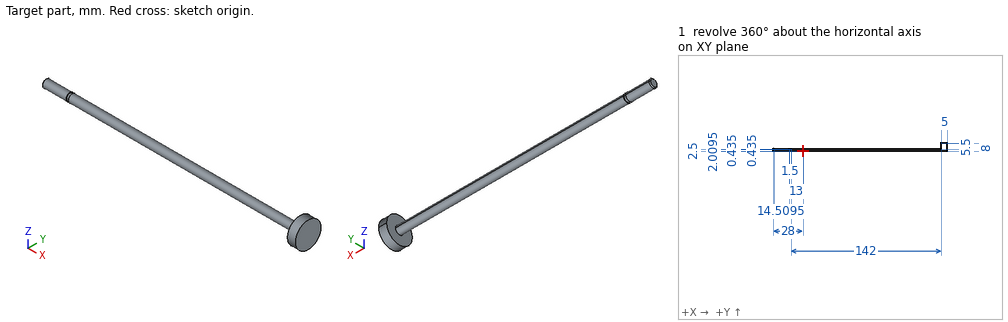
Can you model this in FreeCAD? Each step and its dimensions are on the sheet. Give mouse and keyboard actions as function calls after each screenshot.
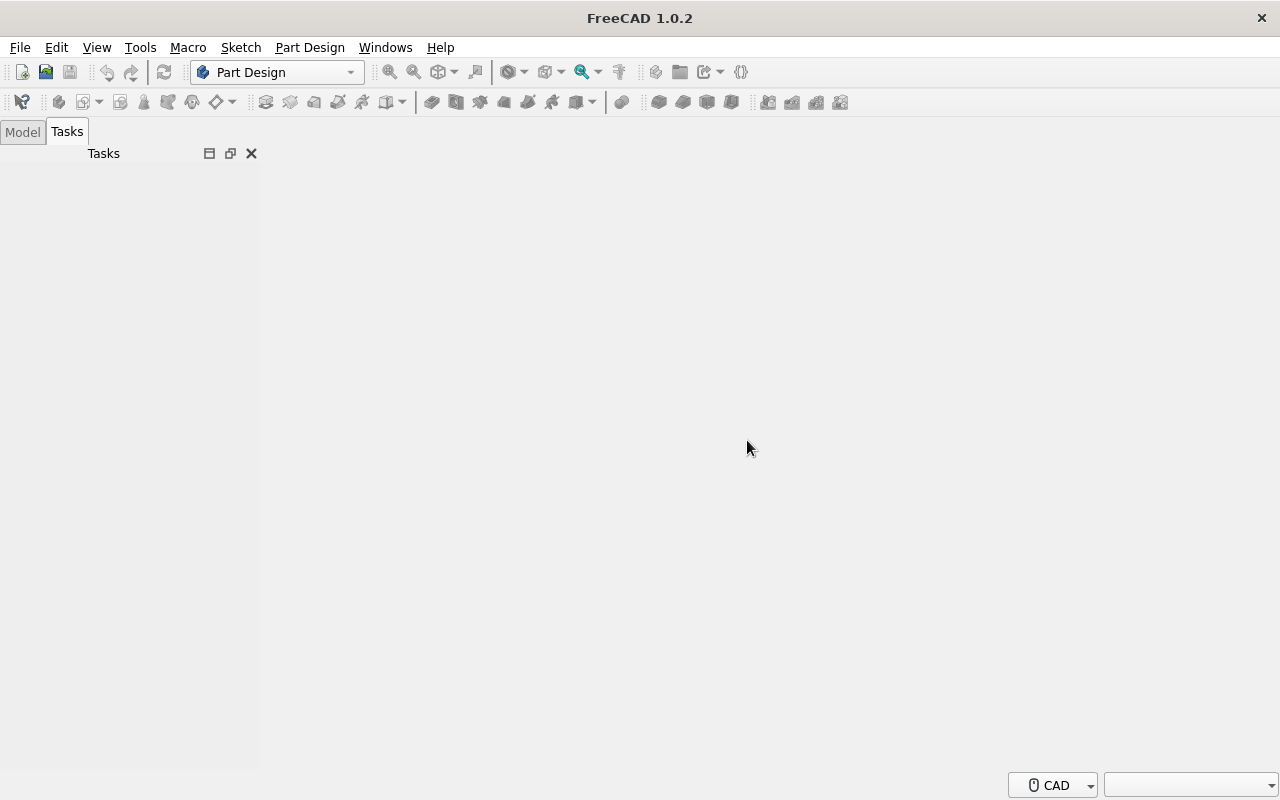
key(ctrl+n)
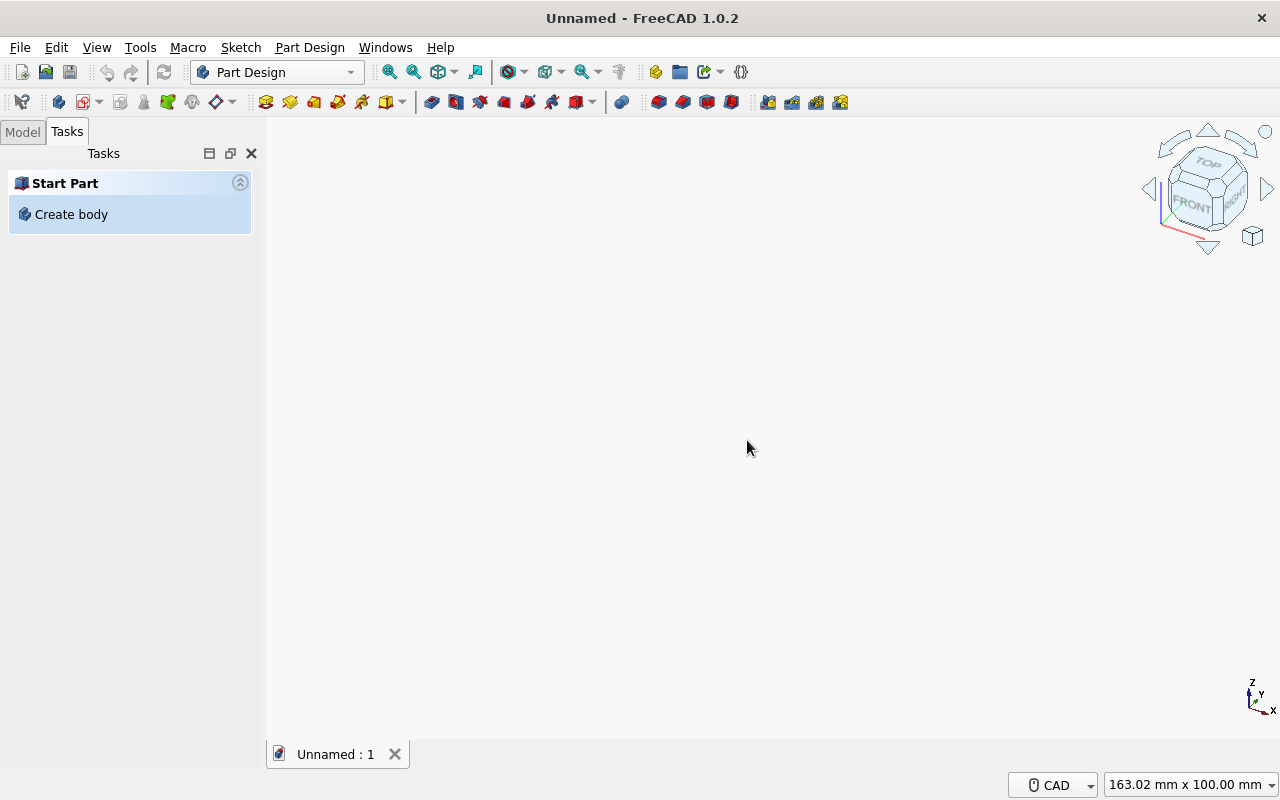
click(84, 102)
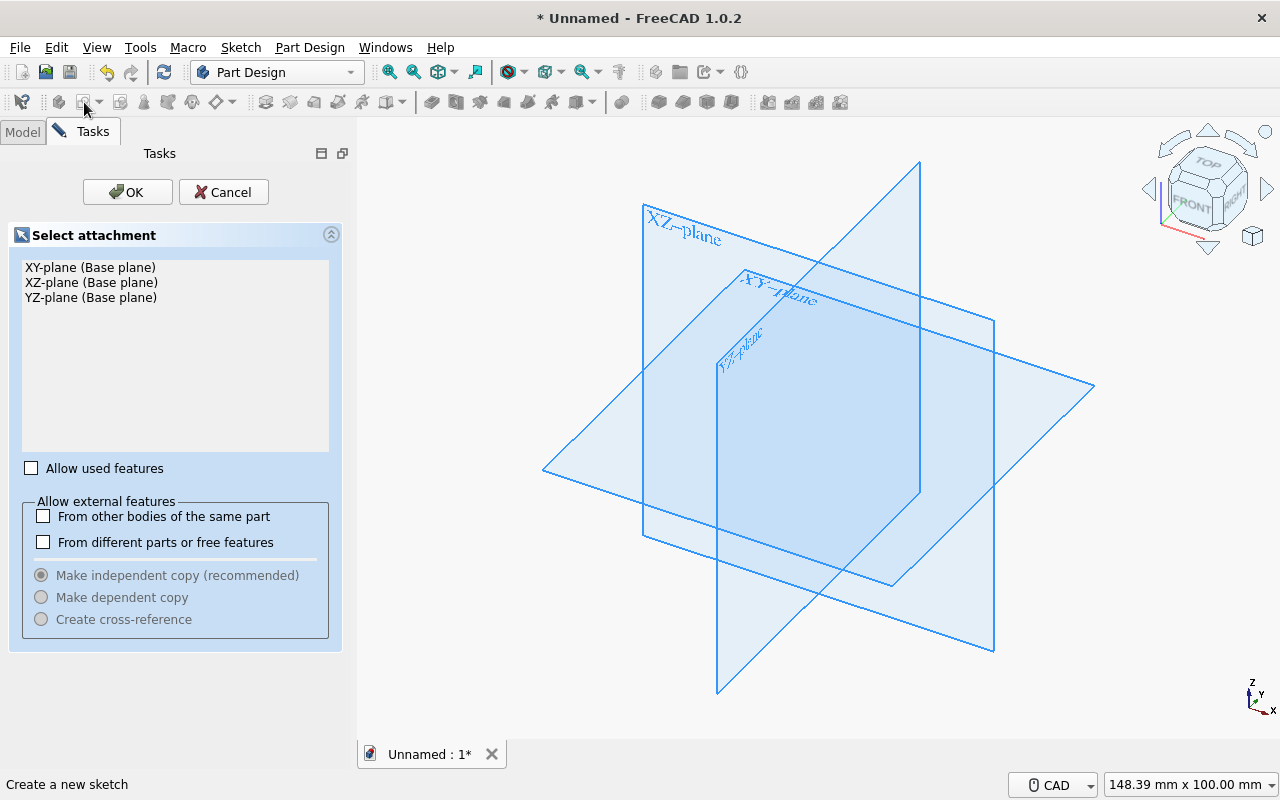
click(82, 268)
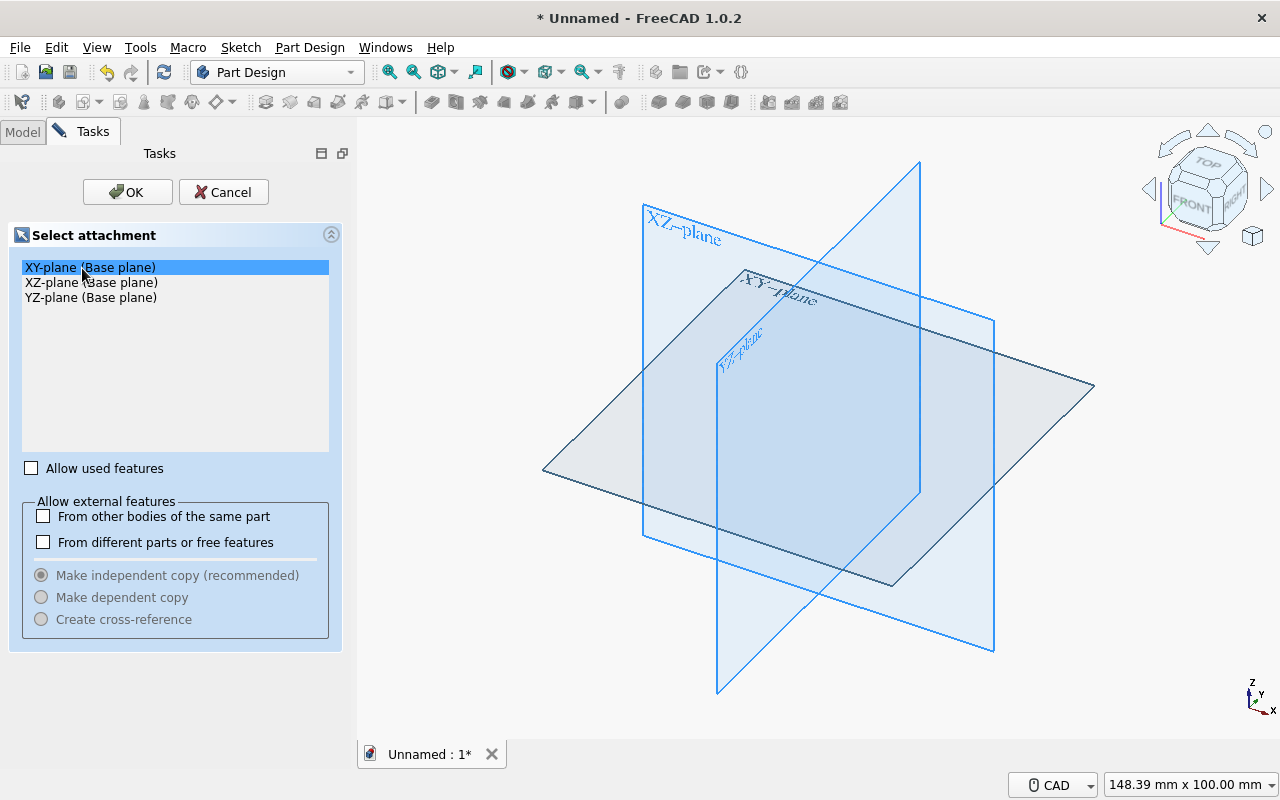
click(128, 192)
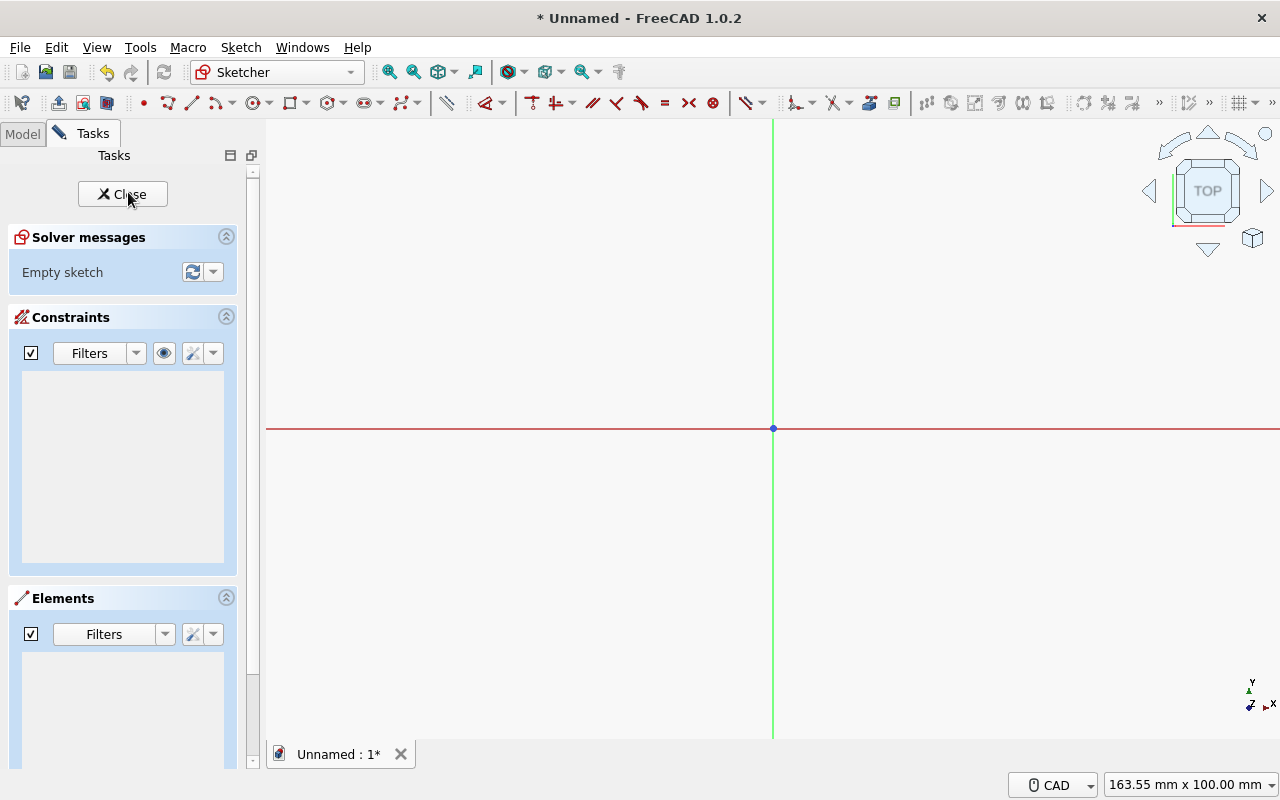
scroll(294, 459, down, 3)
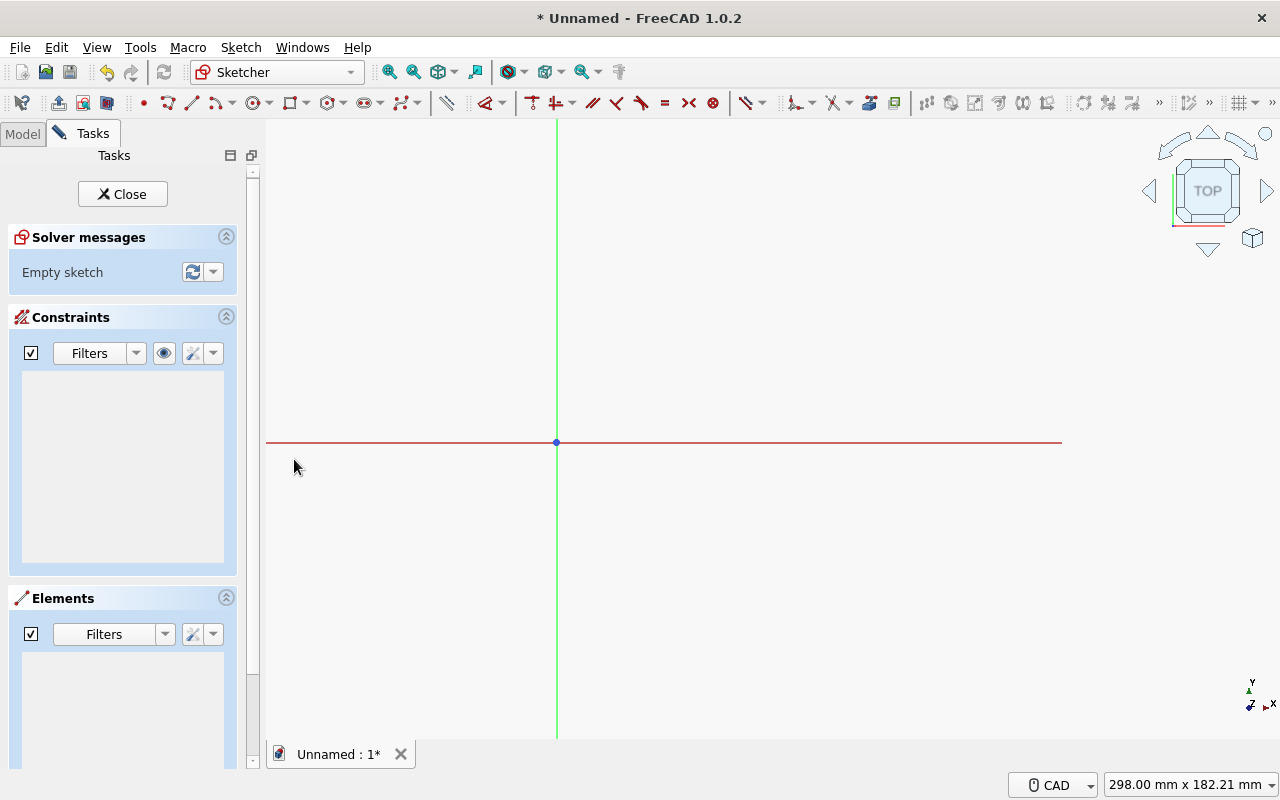
click(168, 104)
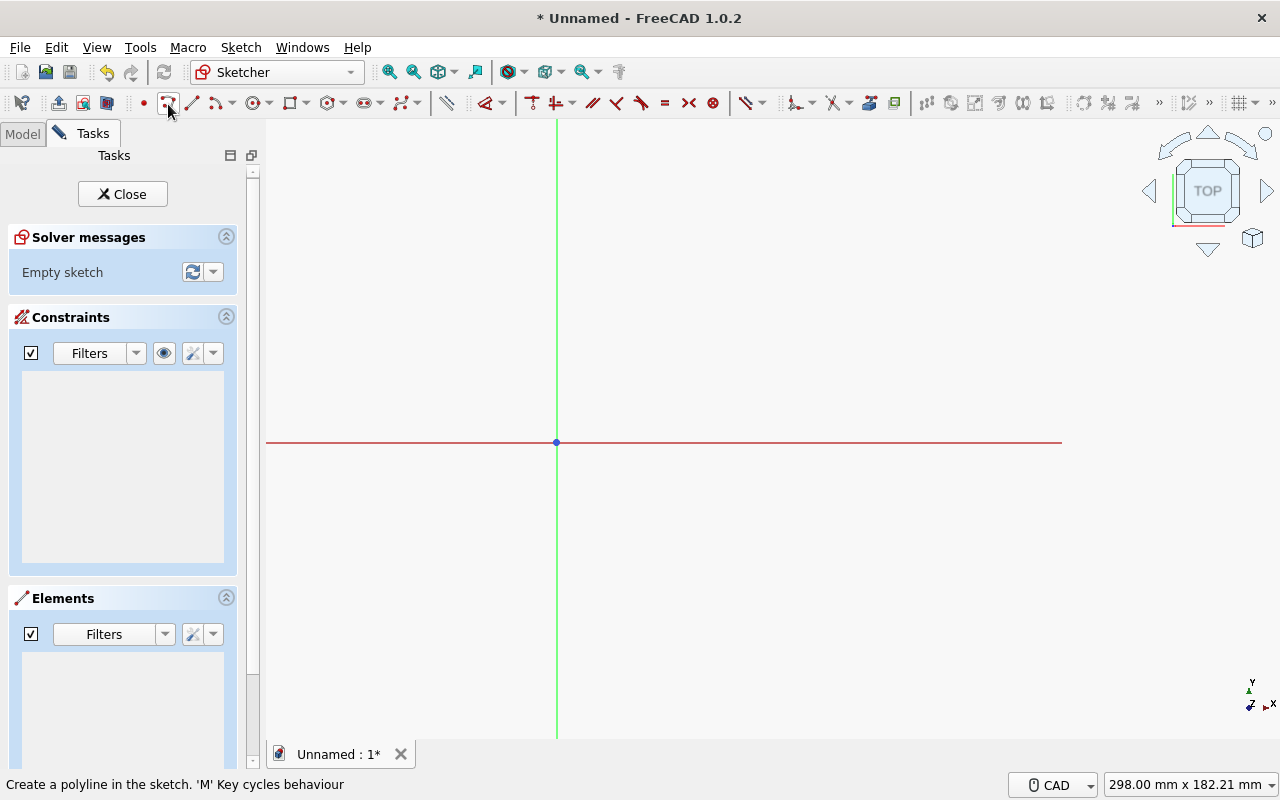
scroll(518, 436, up, 5)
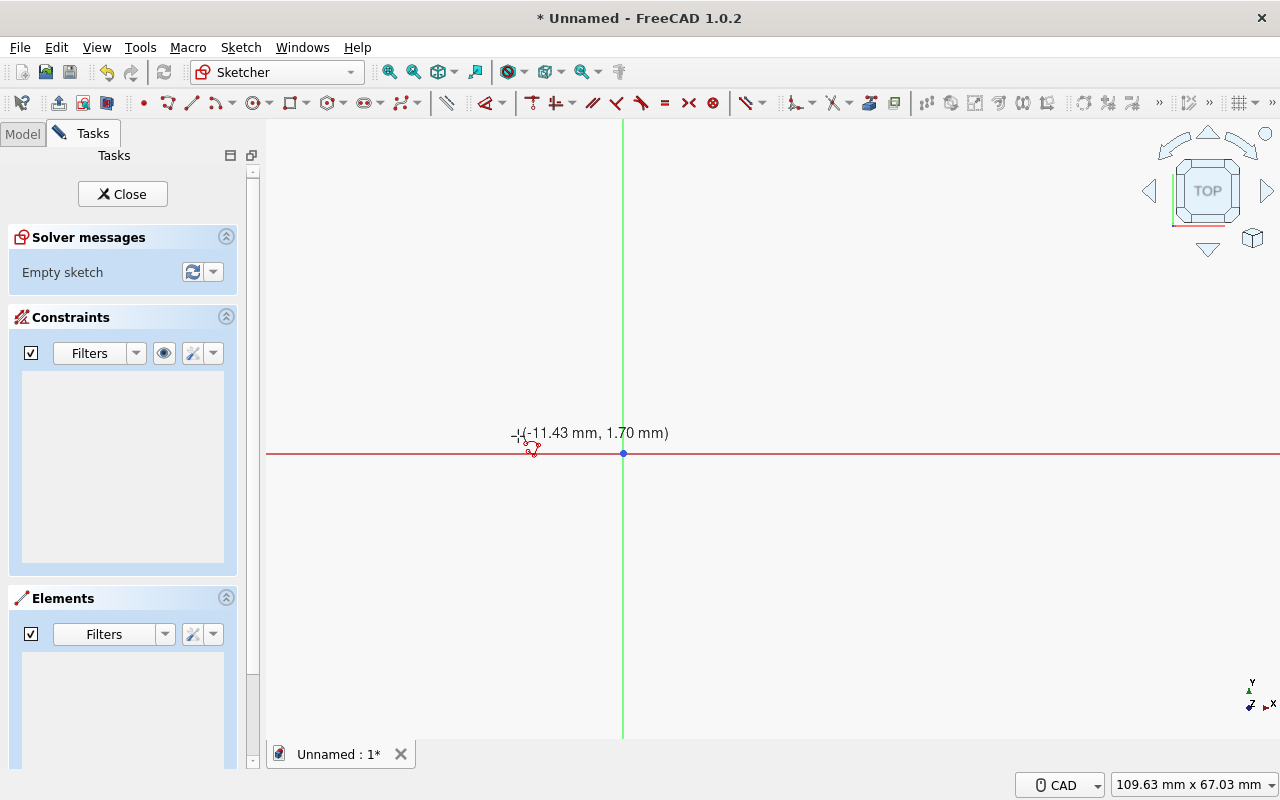
click(517, 434)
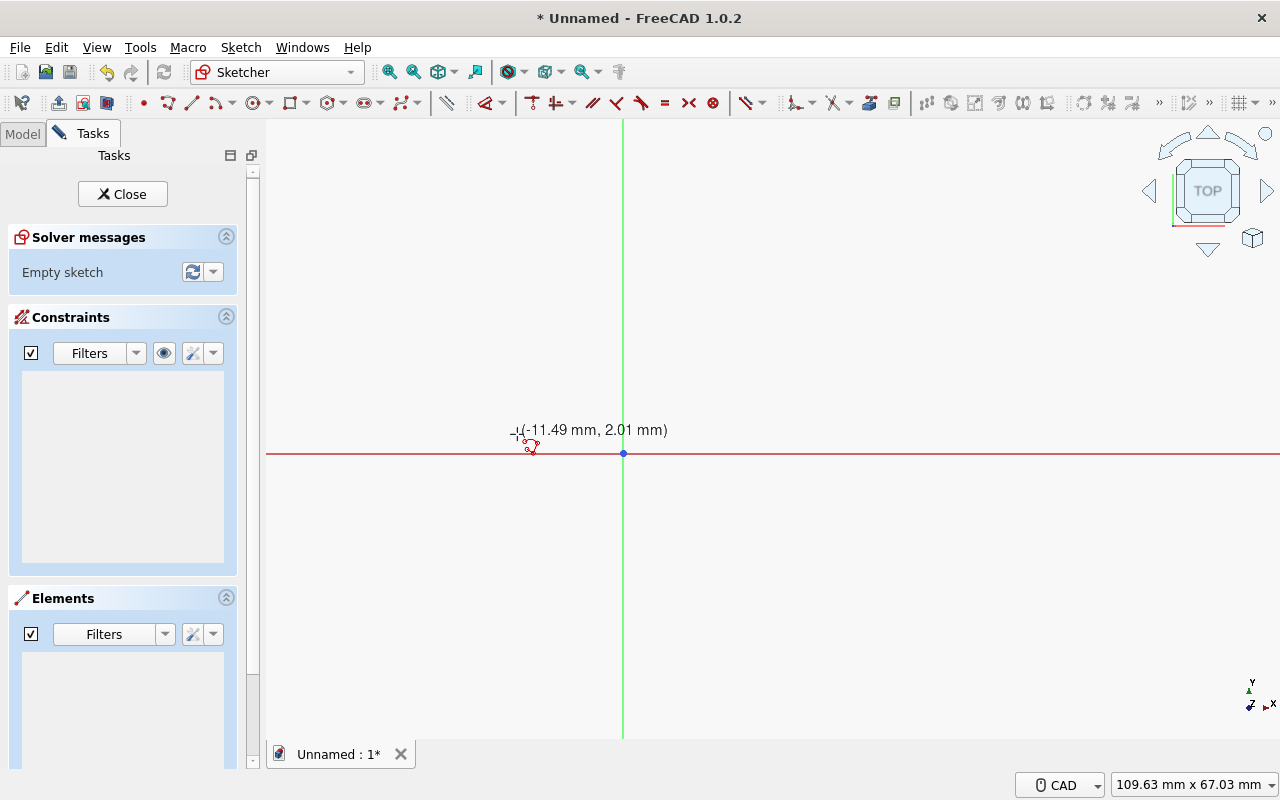
scroll(517, 430, up, 7)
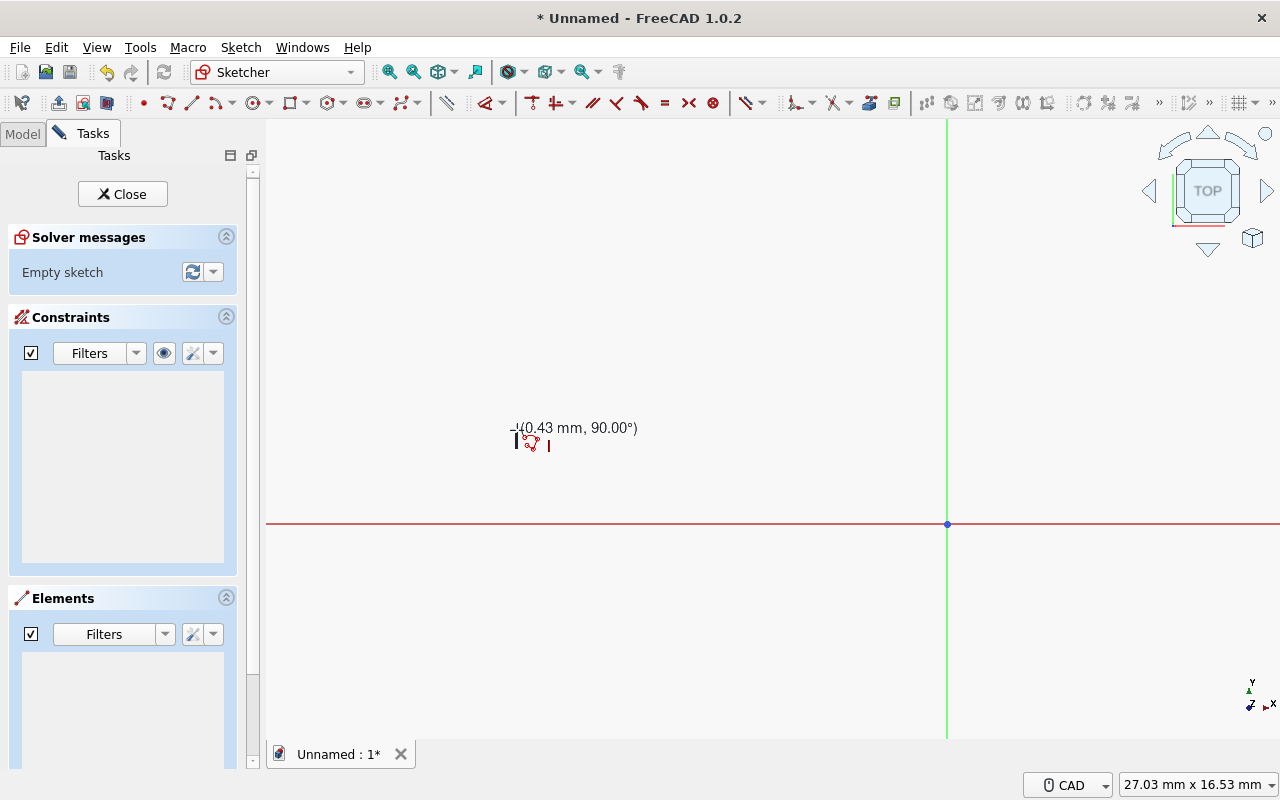
click(516, 430)